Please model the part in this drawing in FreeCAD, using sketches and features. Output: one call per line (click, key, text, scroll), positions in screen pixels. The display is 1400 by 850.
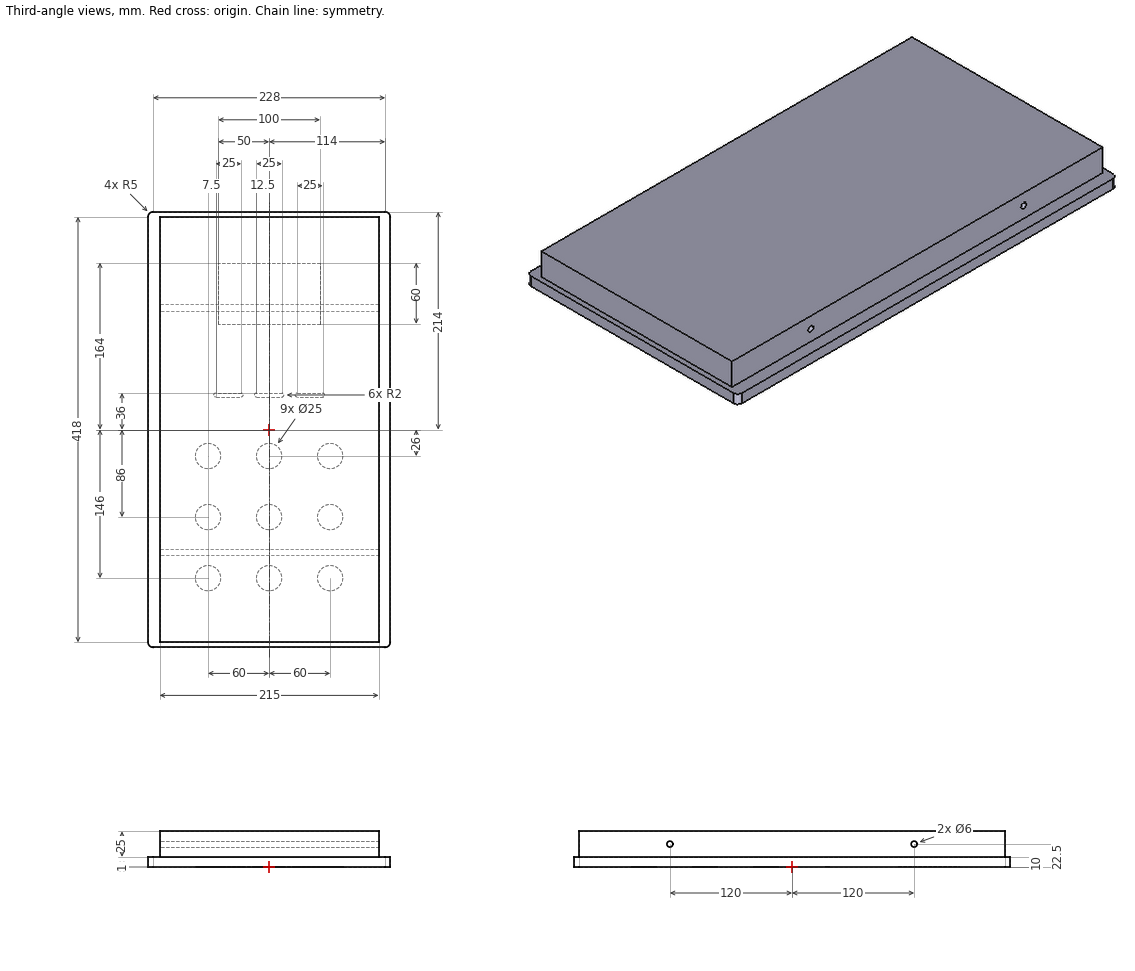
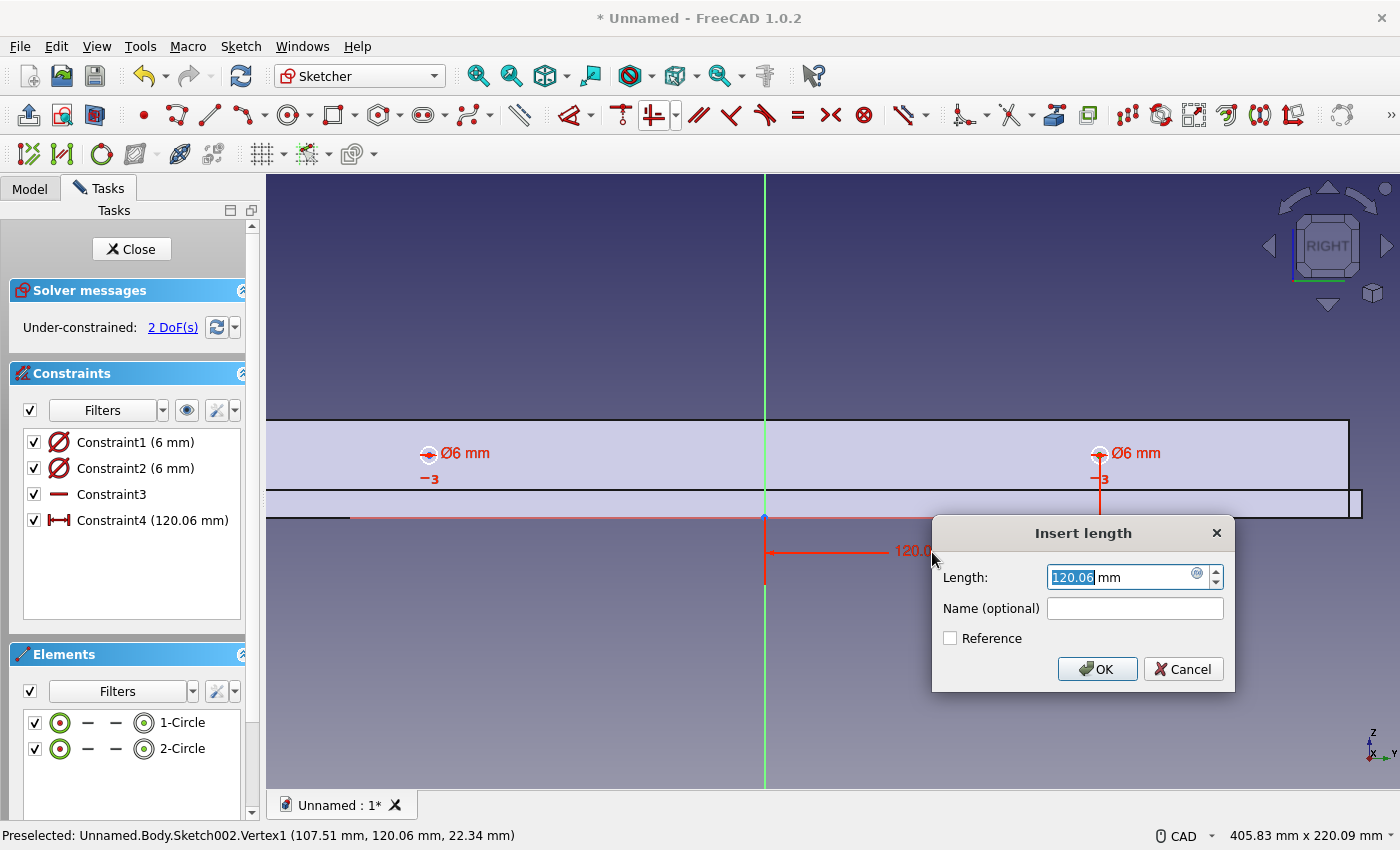
text(120)
key(Return)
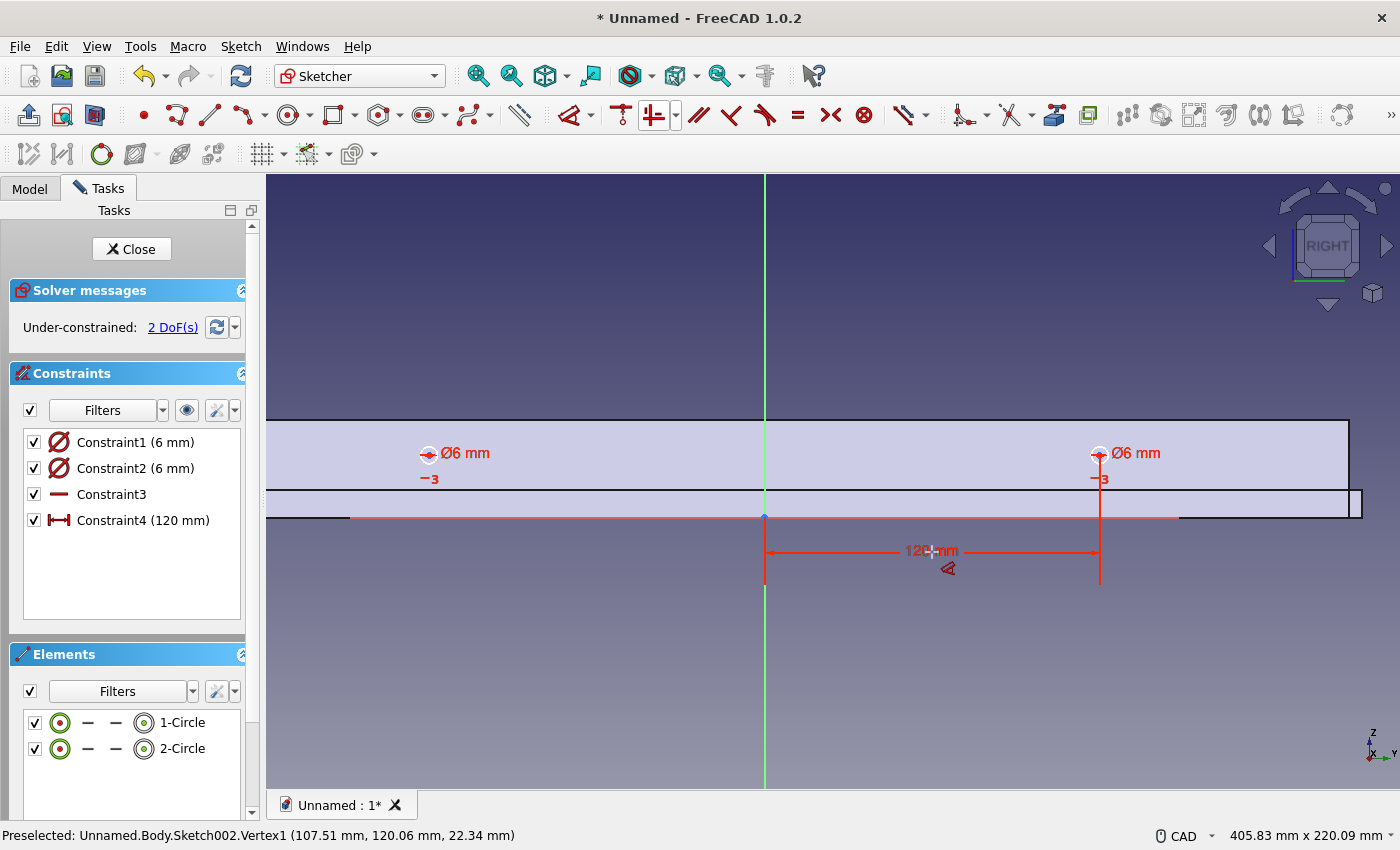
click(429, 455)
click(597, 552)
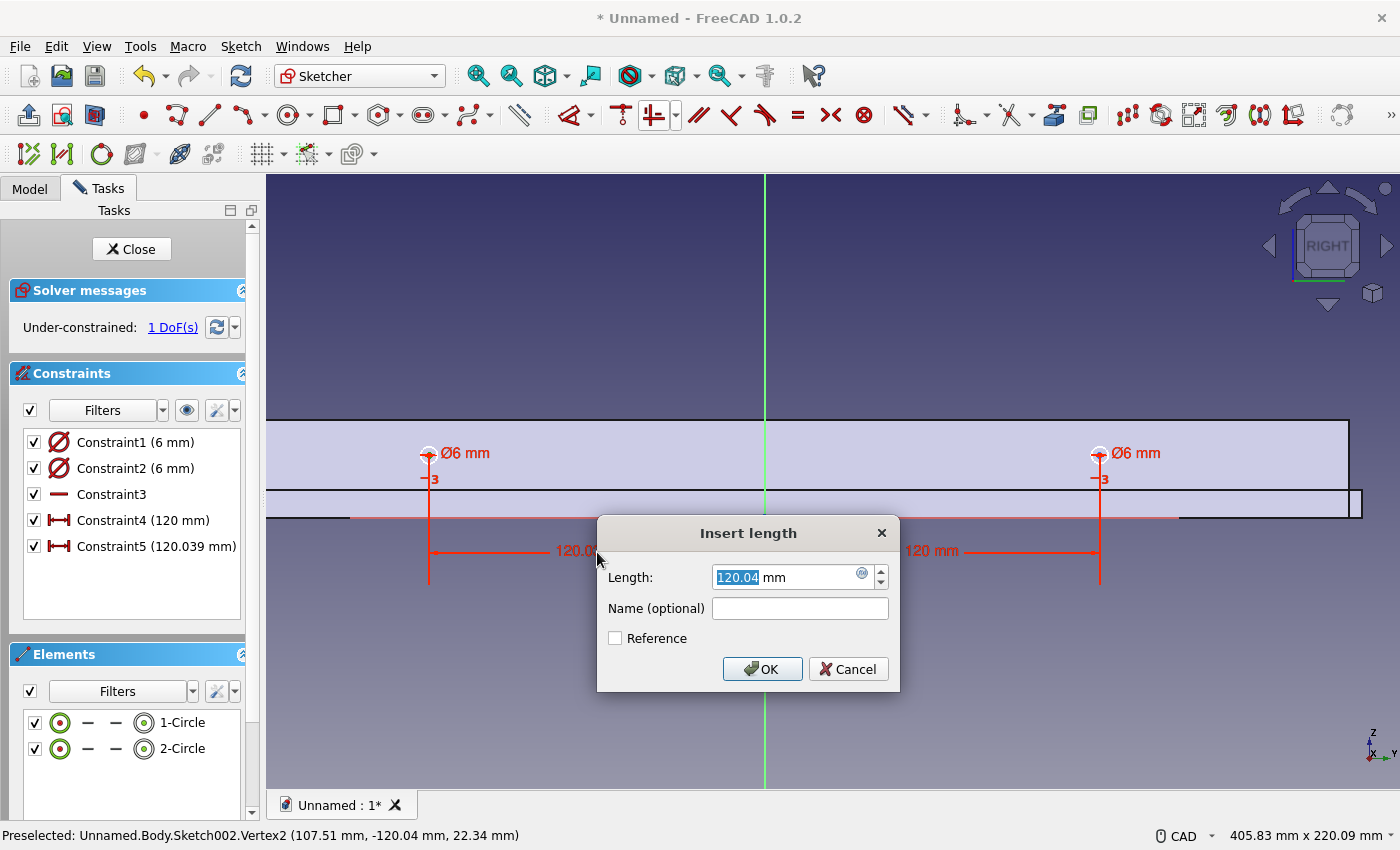
text(120)
key(Return)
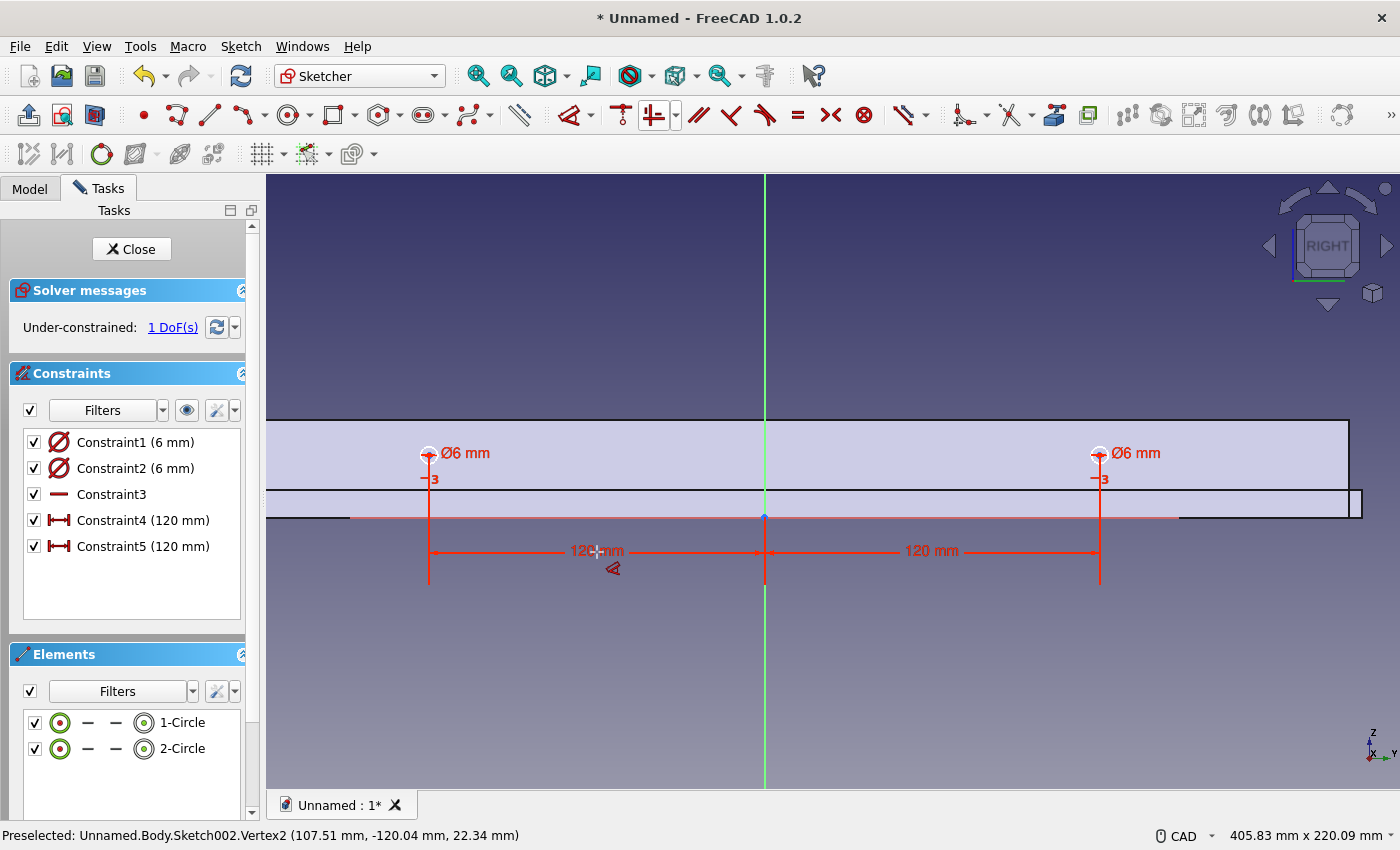
click(1100, 455)
click(1134, 487)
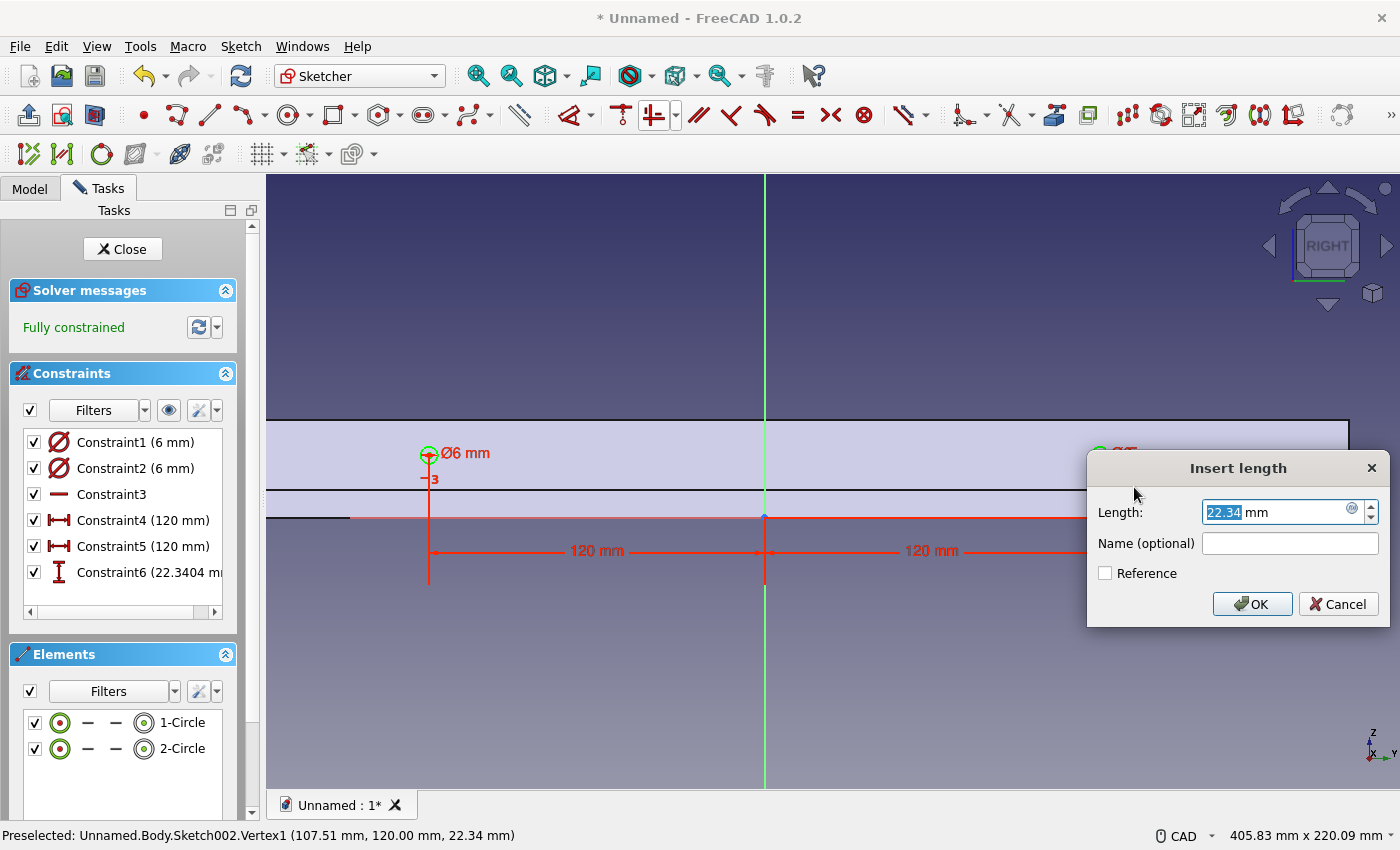
text(22.5)
key(Return)
key(Escape)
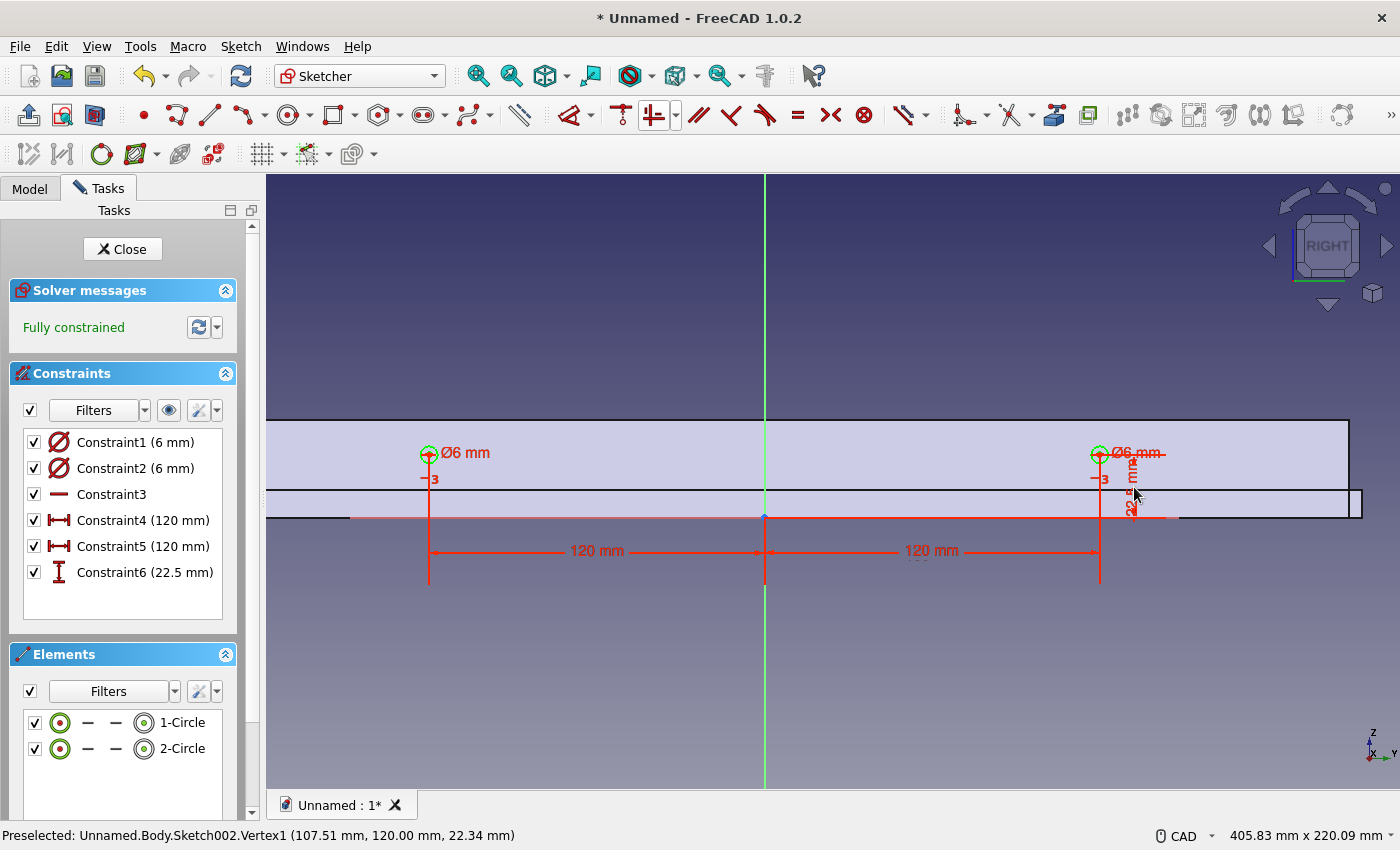
click(123, 249)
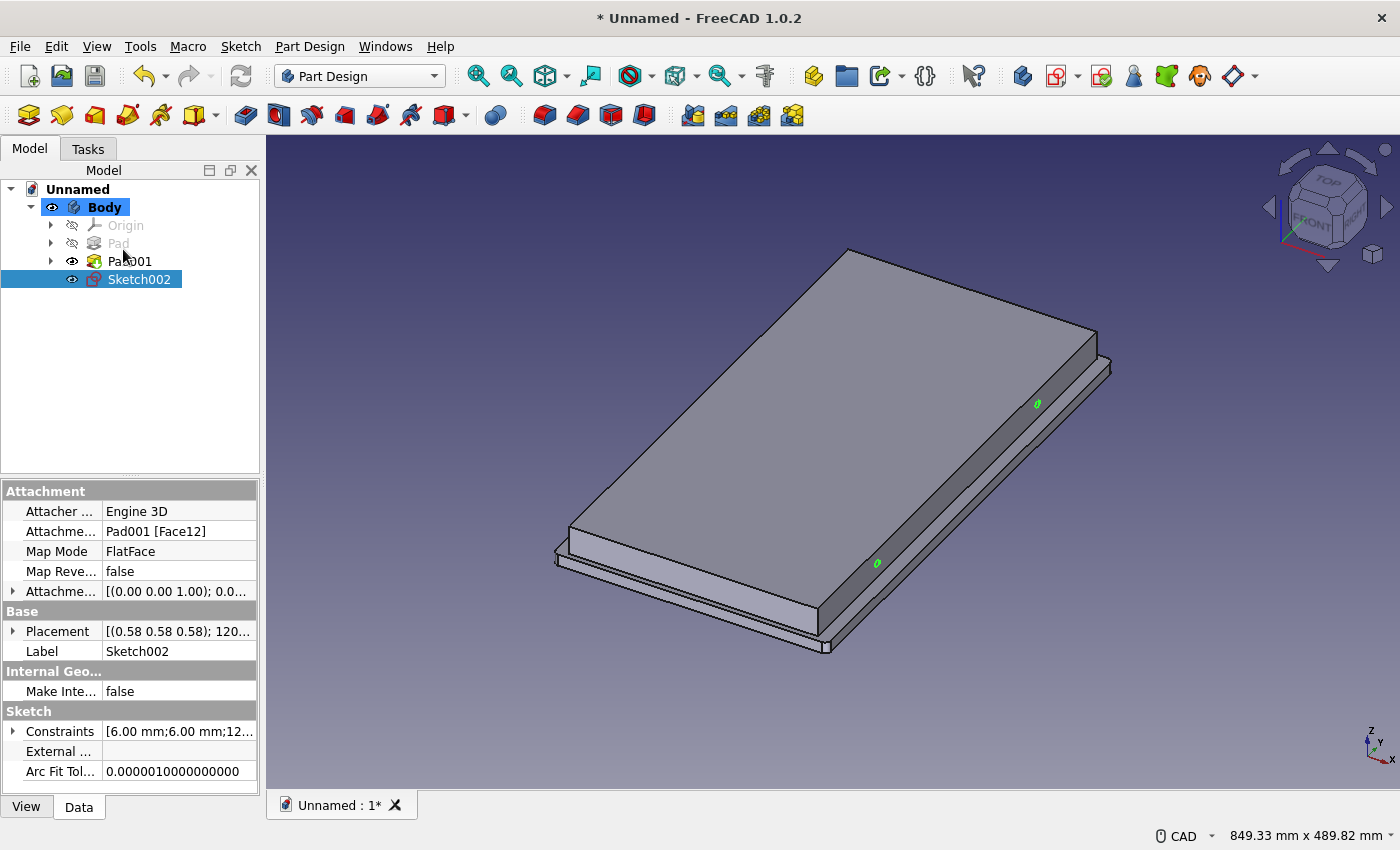
click(246, 116)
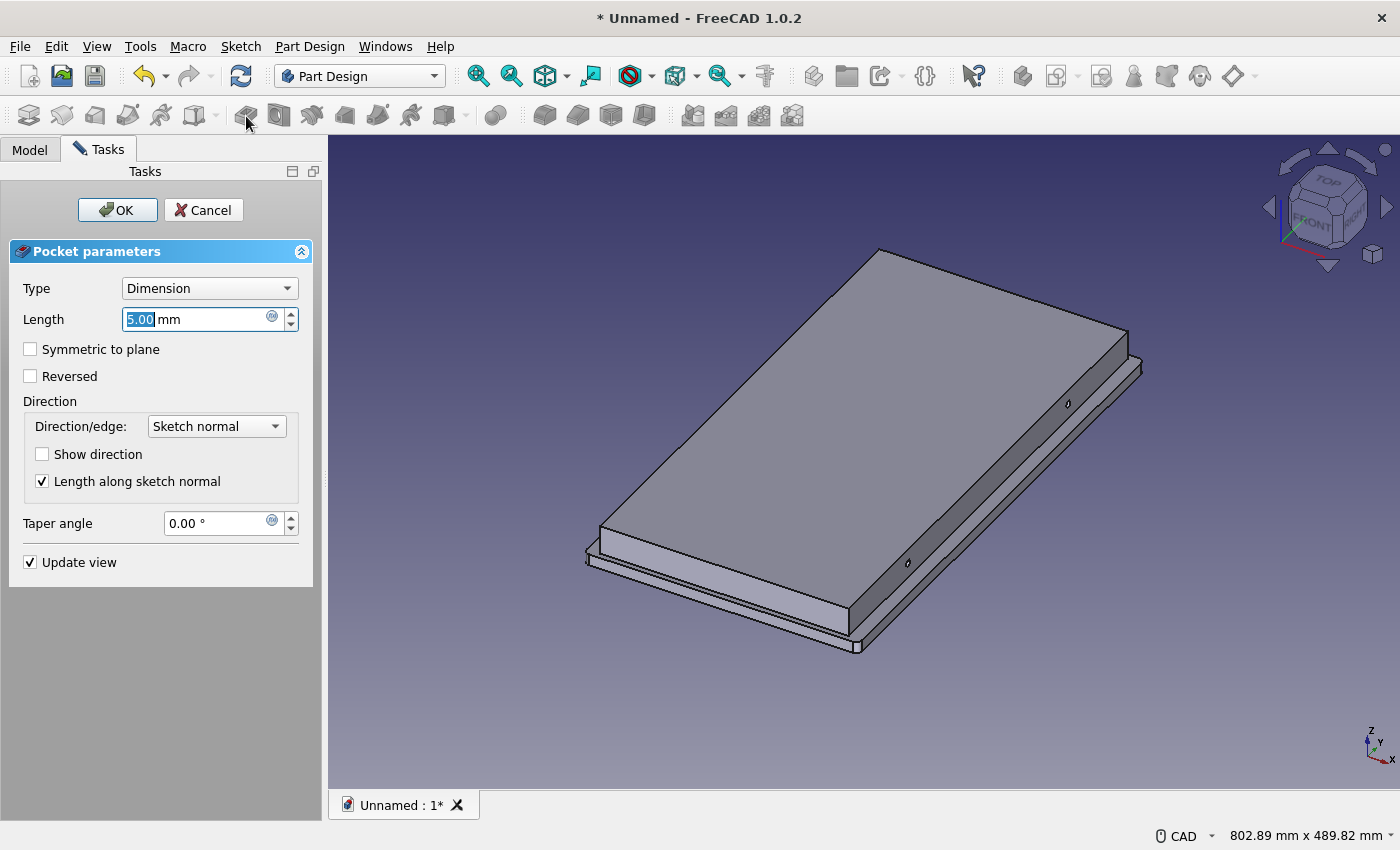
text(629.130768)
key(Tab)